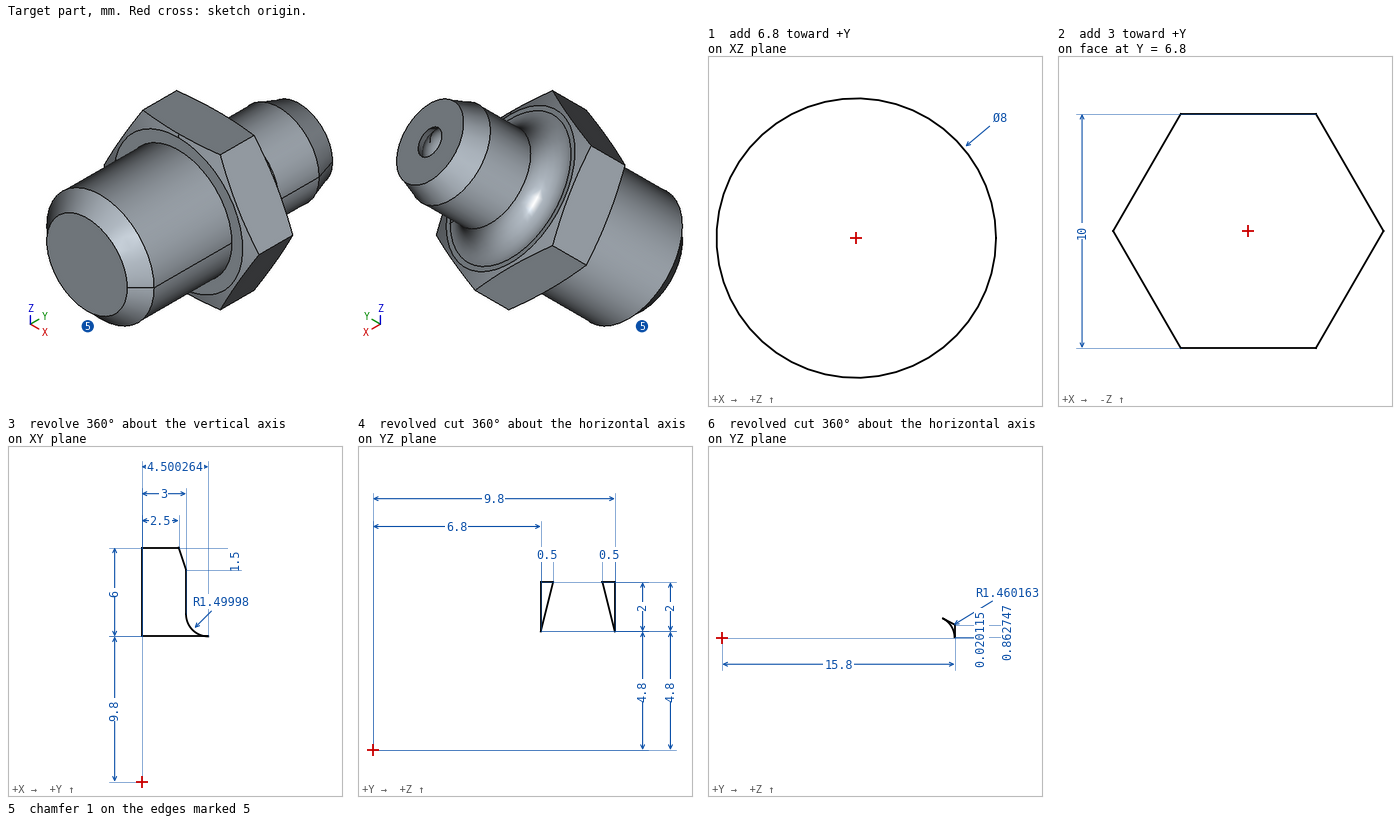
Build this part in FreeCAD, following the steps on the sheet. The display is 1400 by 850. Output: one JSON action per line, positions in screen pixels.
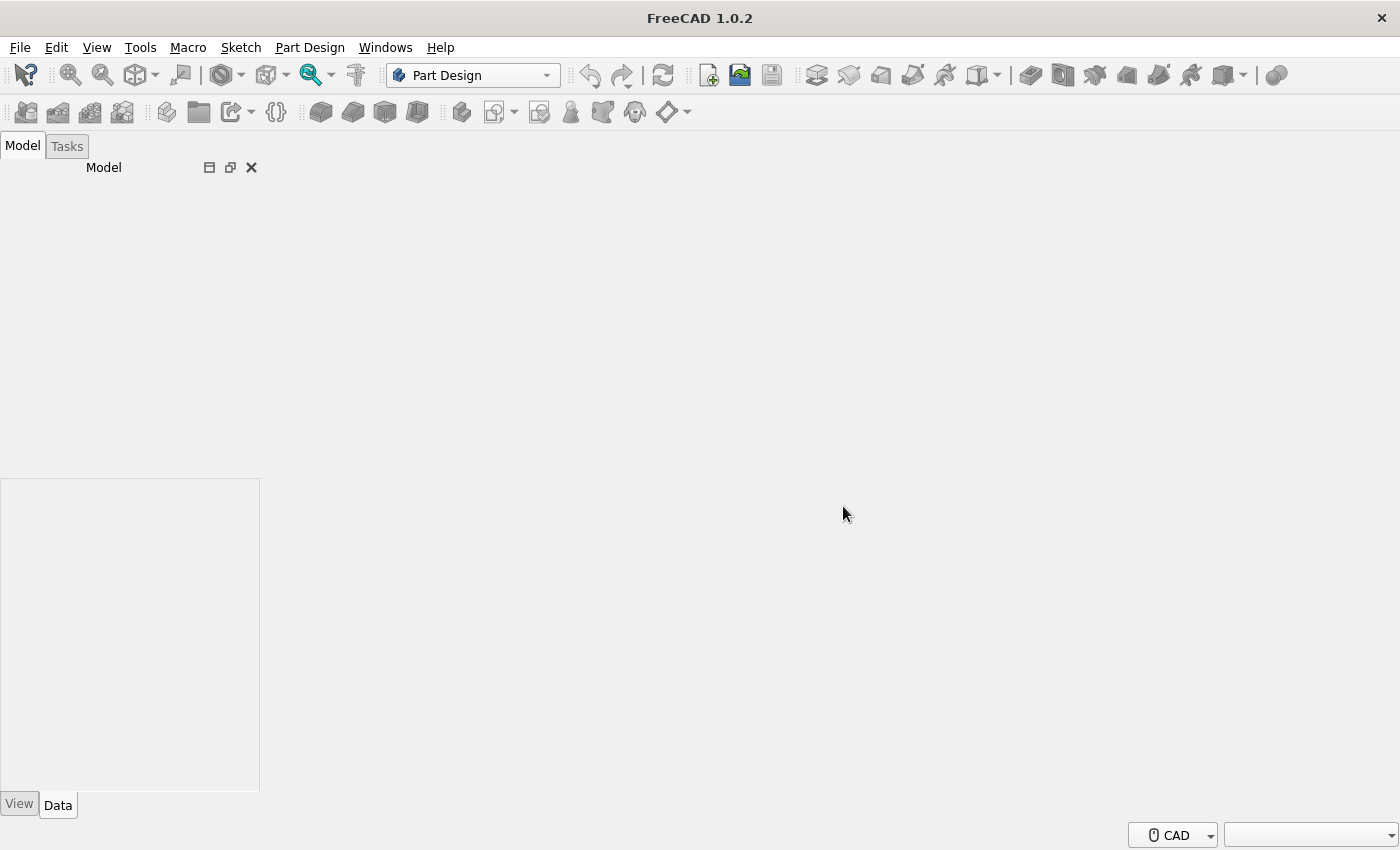
{"action": "key", "text": "ctrl+n"}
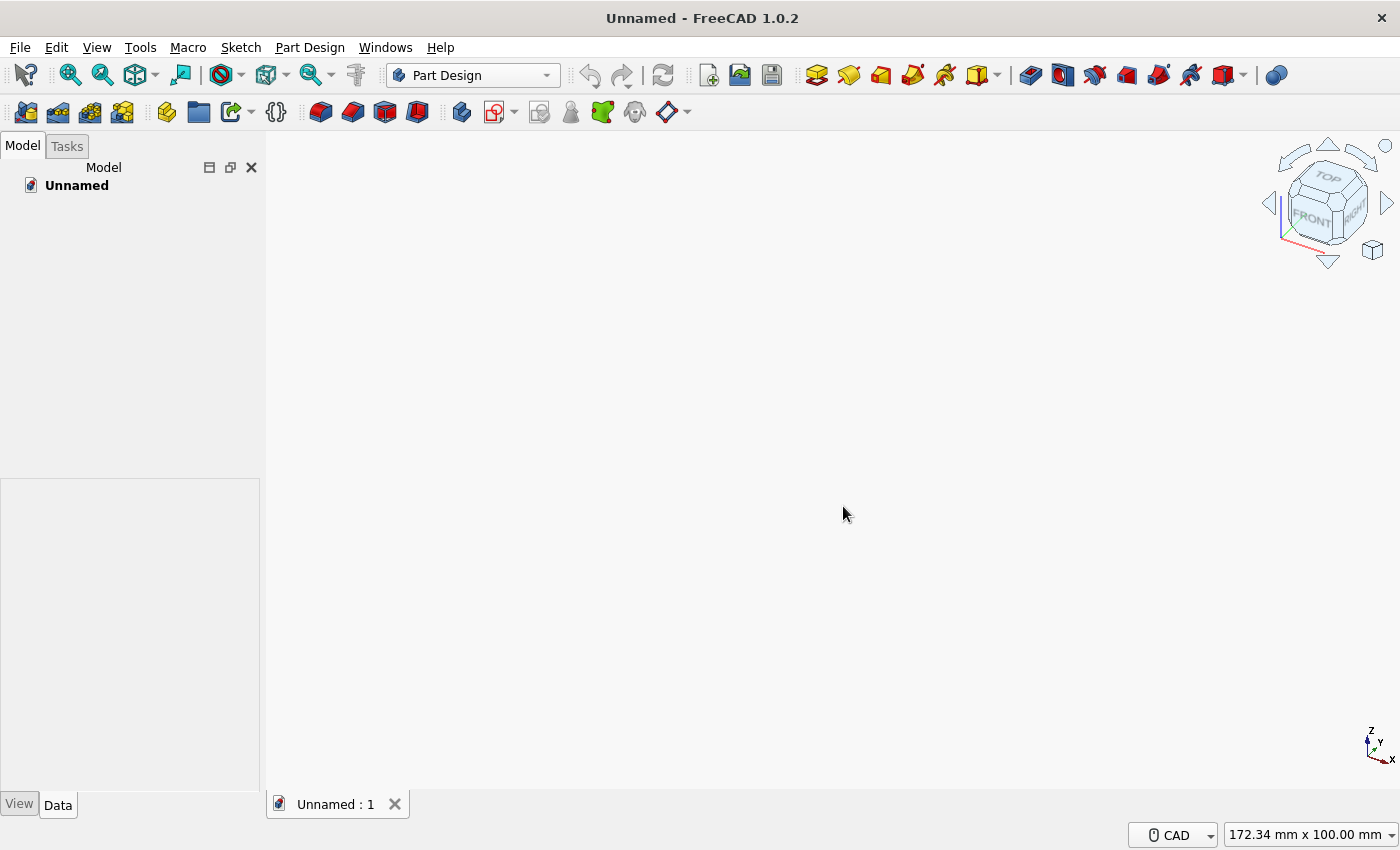
{"action": "left_click", "coordinate": [494, 112]}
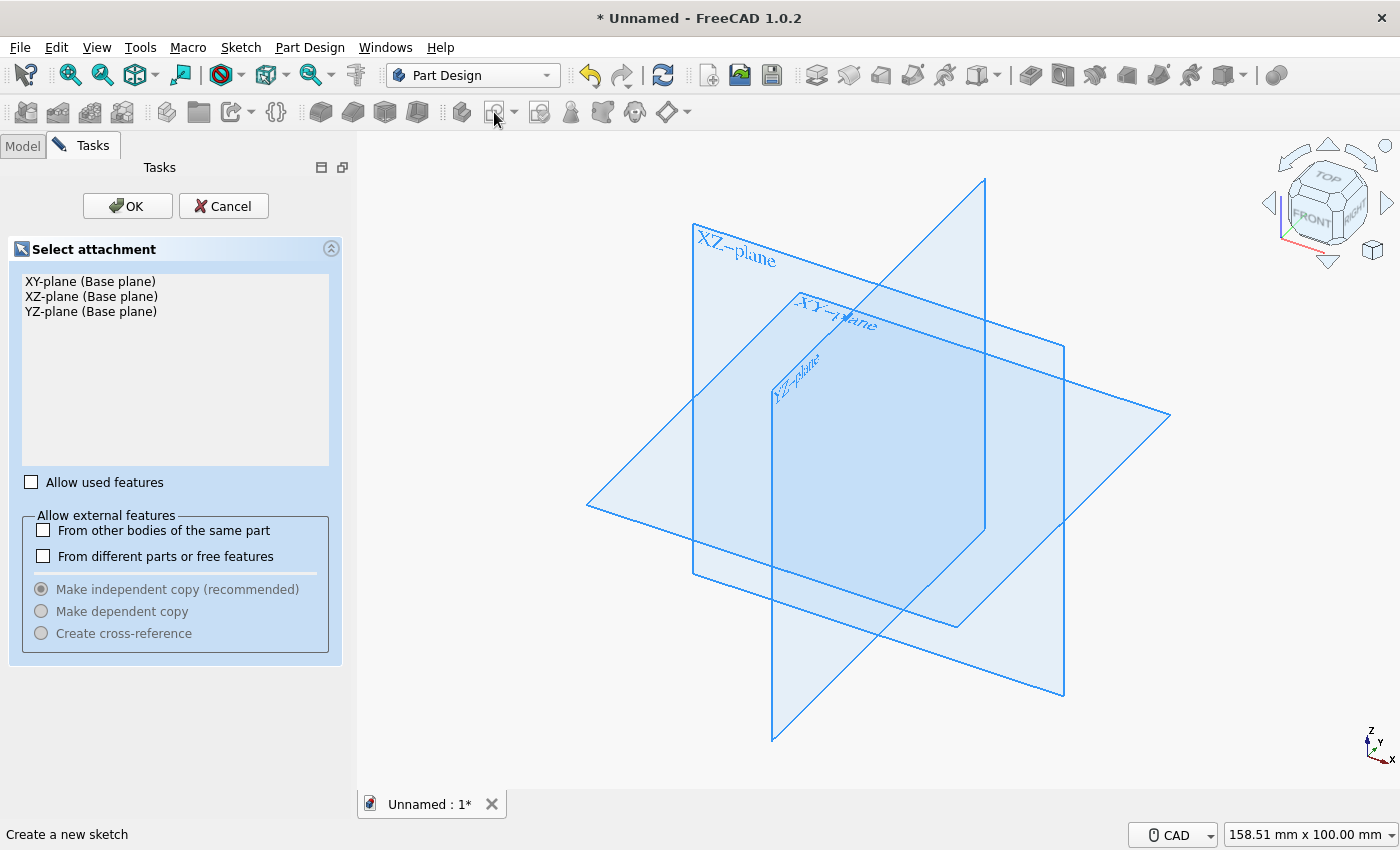
{"action": "left_click", "coordinate": [82, 296]}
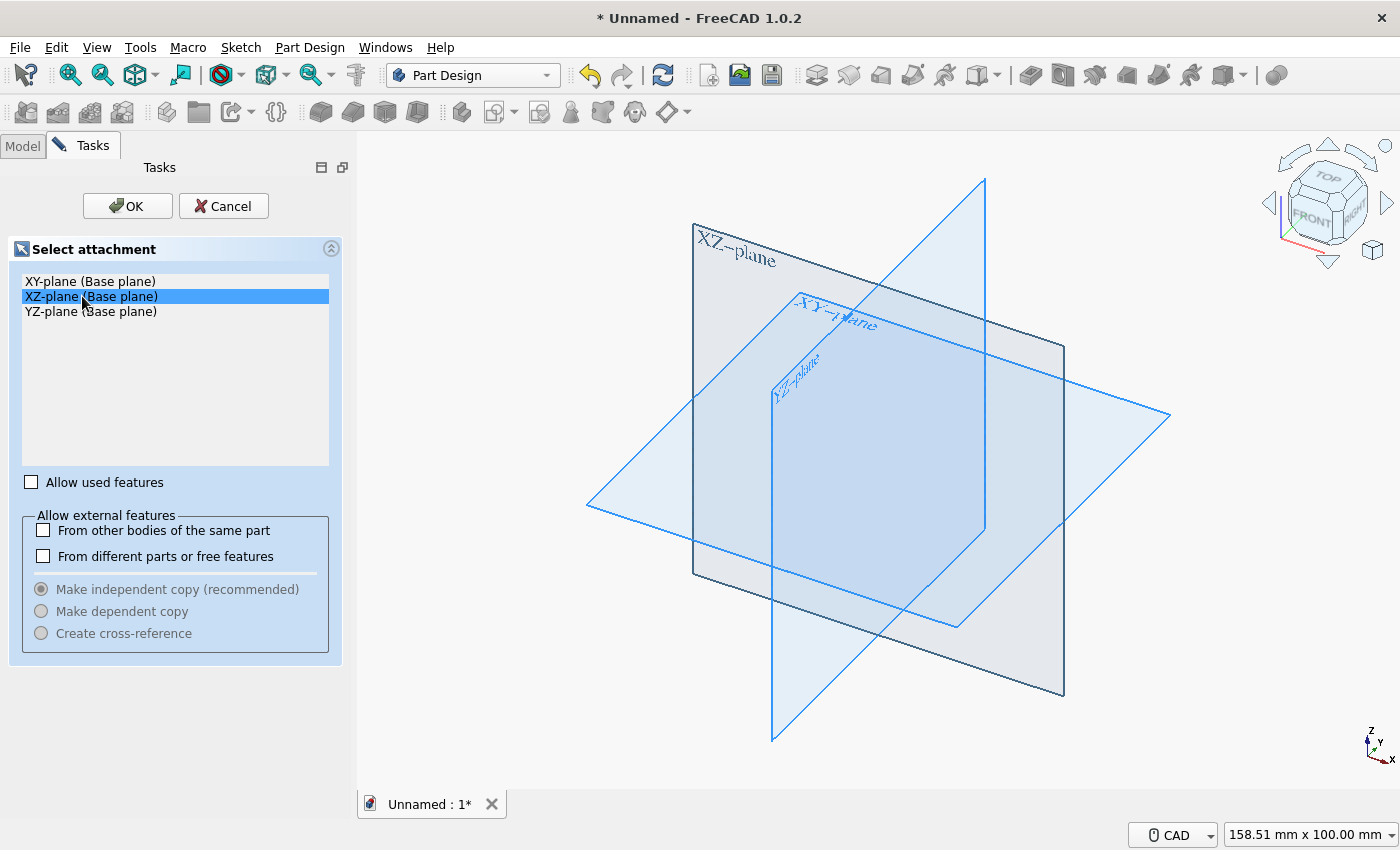
{"action": "left_click", "coordinate": [128, 206]}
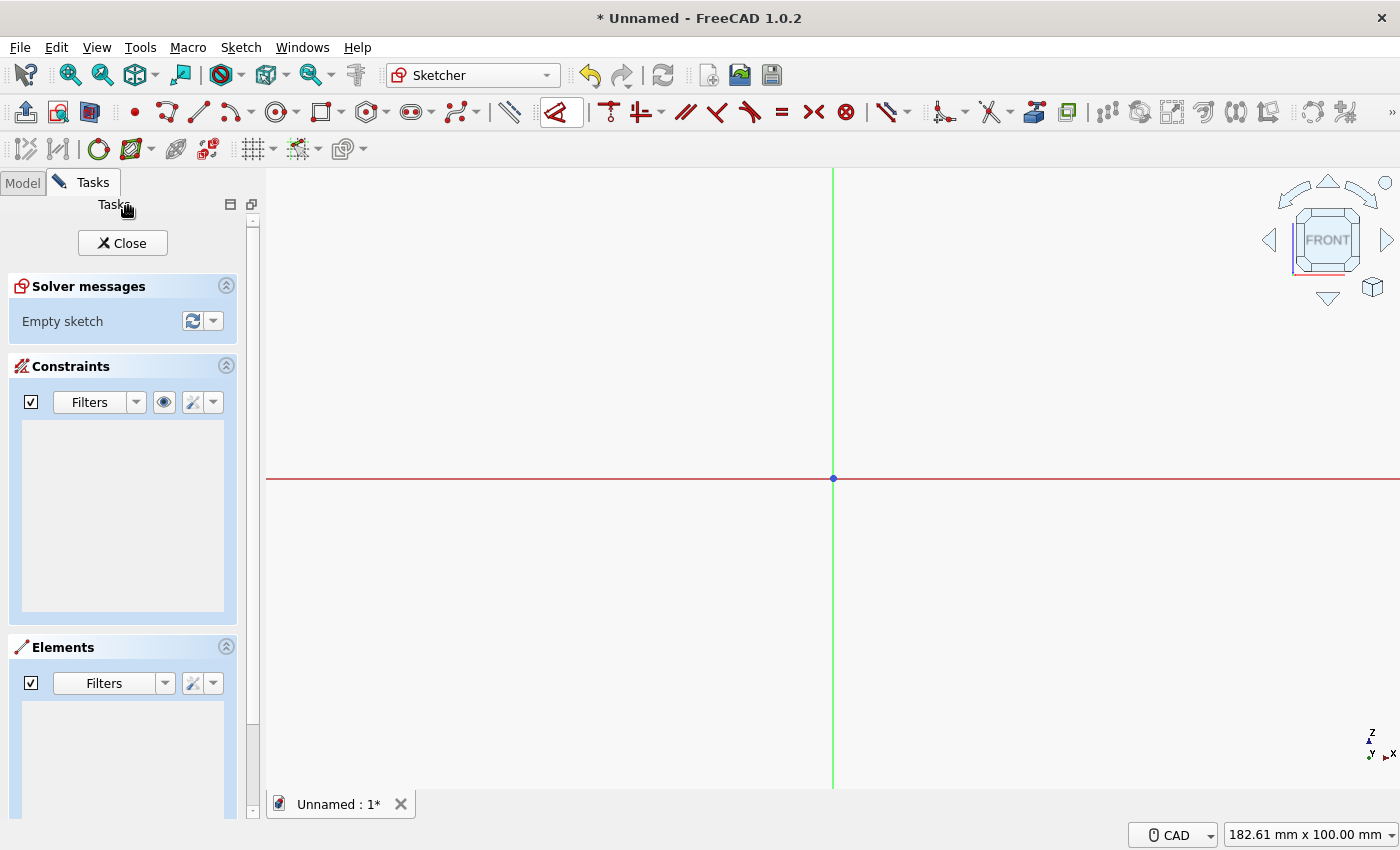
{"action": "scroll", "coordinate": [844, 478], "scroll_direction": "up", "scroll_amount": 10}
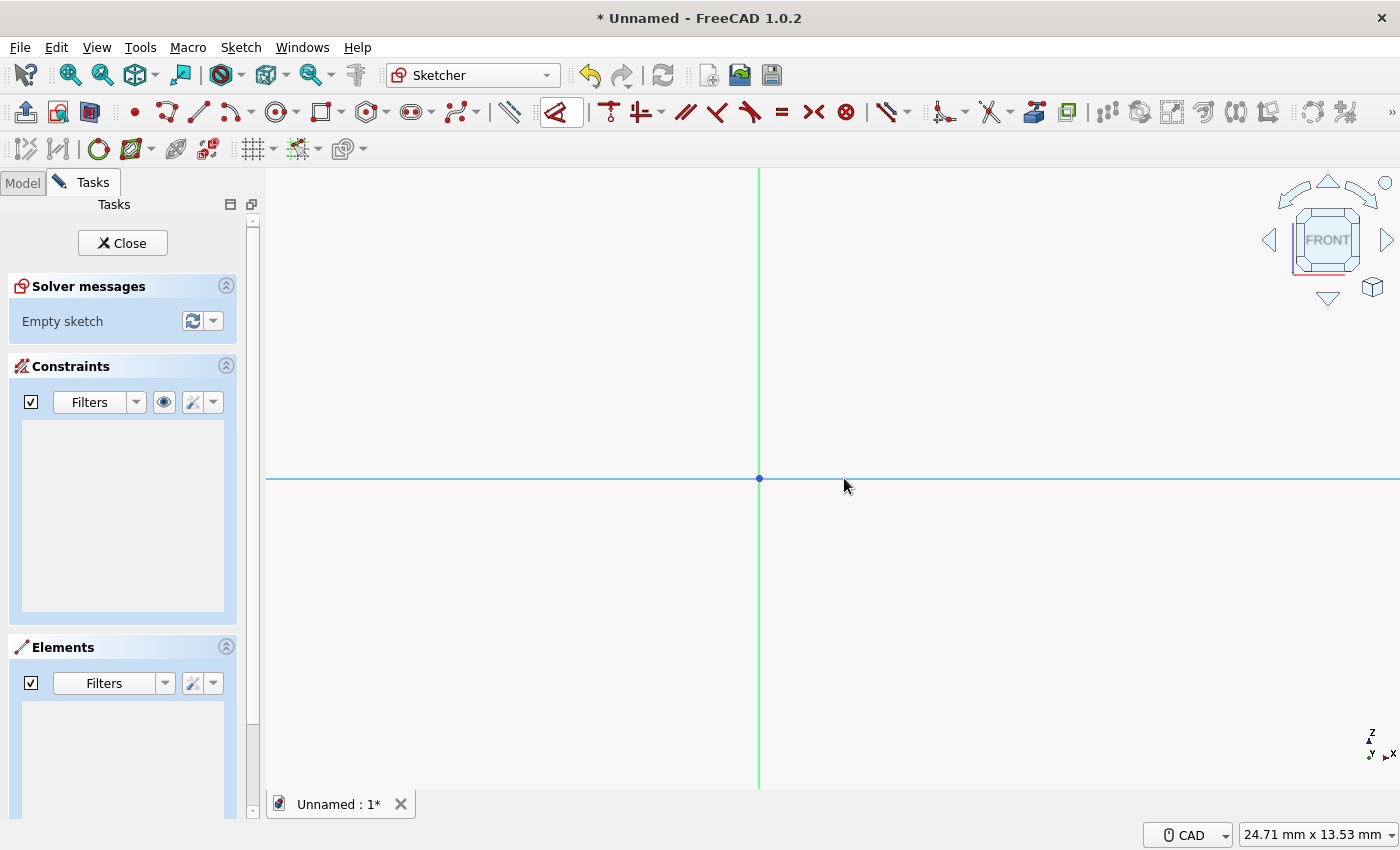
{"action": "key", "text": "g c"}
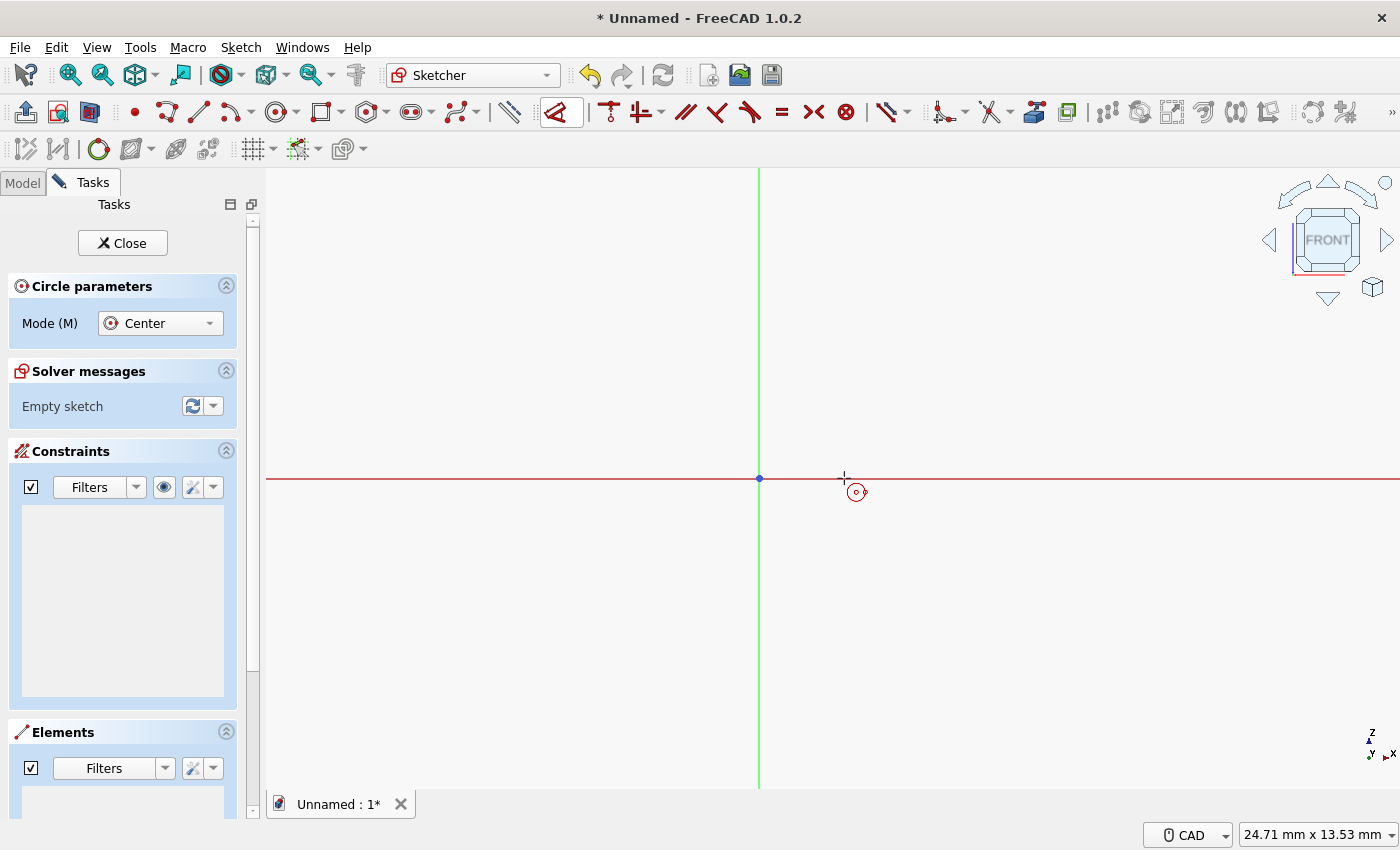
{"action": "left_click", "coordinate": [759, 478]}
{"action": "mouse_move", "coordinate": [889, 349]}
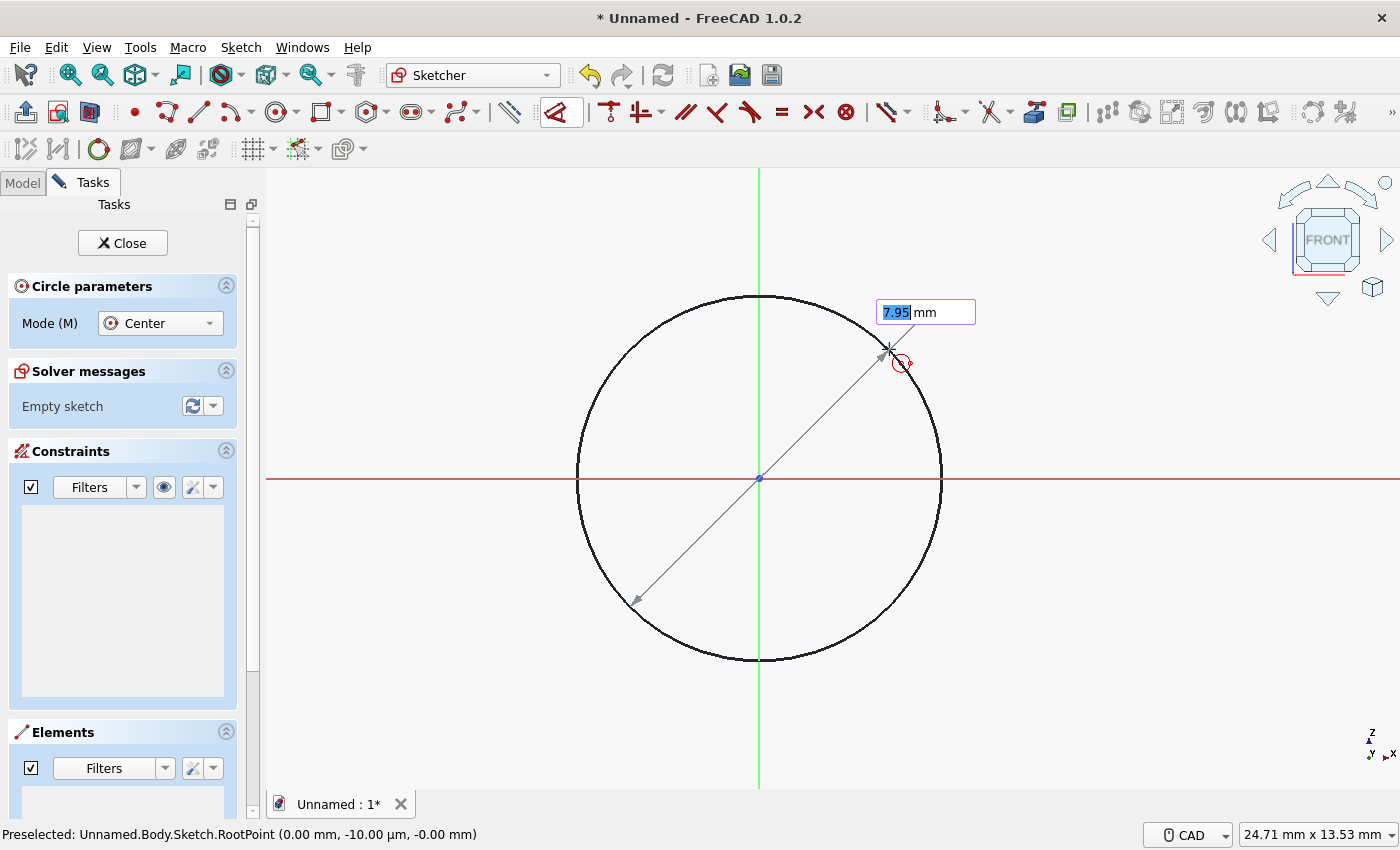
{"action": "type", "text": "8"}
{"action": "key", "text": "Return"}
{"action": "key", "text": "Escape"}